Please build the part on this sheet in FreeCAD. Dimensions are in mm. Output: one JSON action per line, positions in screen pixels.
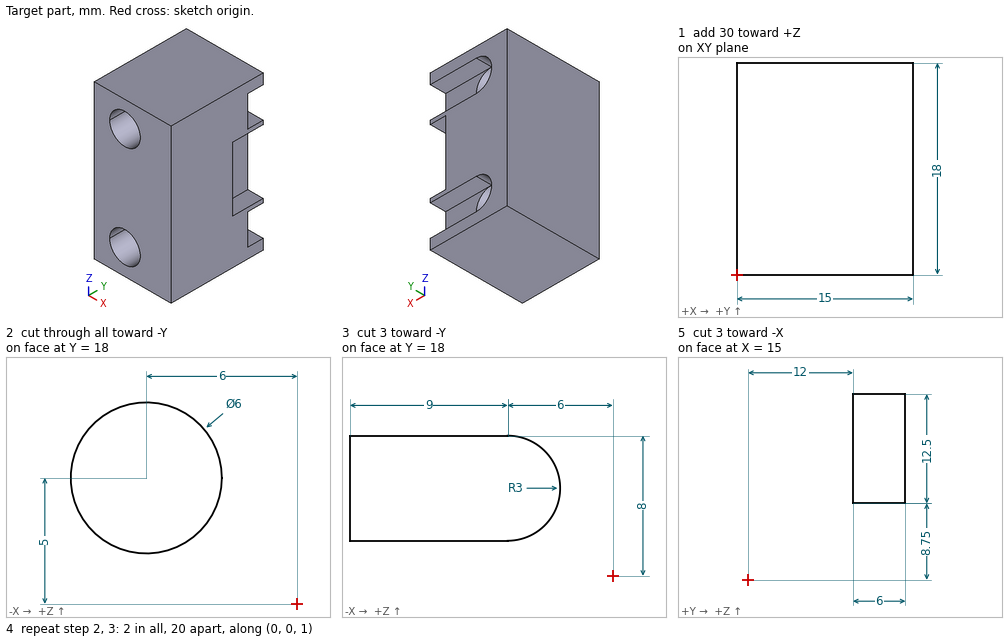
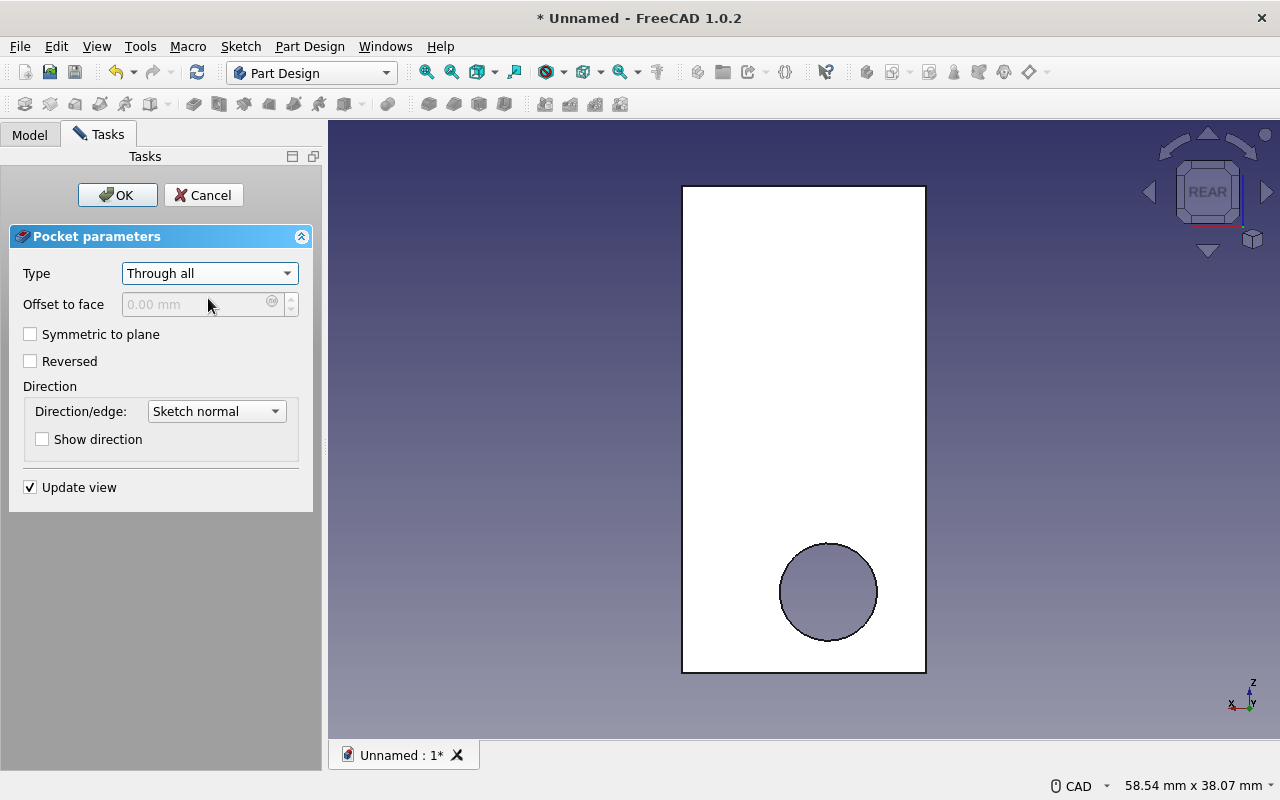
{"action": "left_click", "coordinate": [118, 195]}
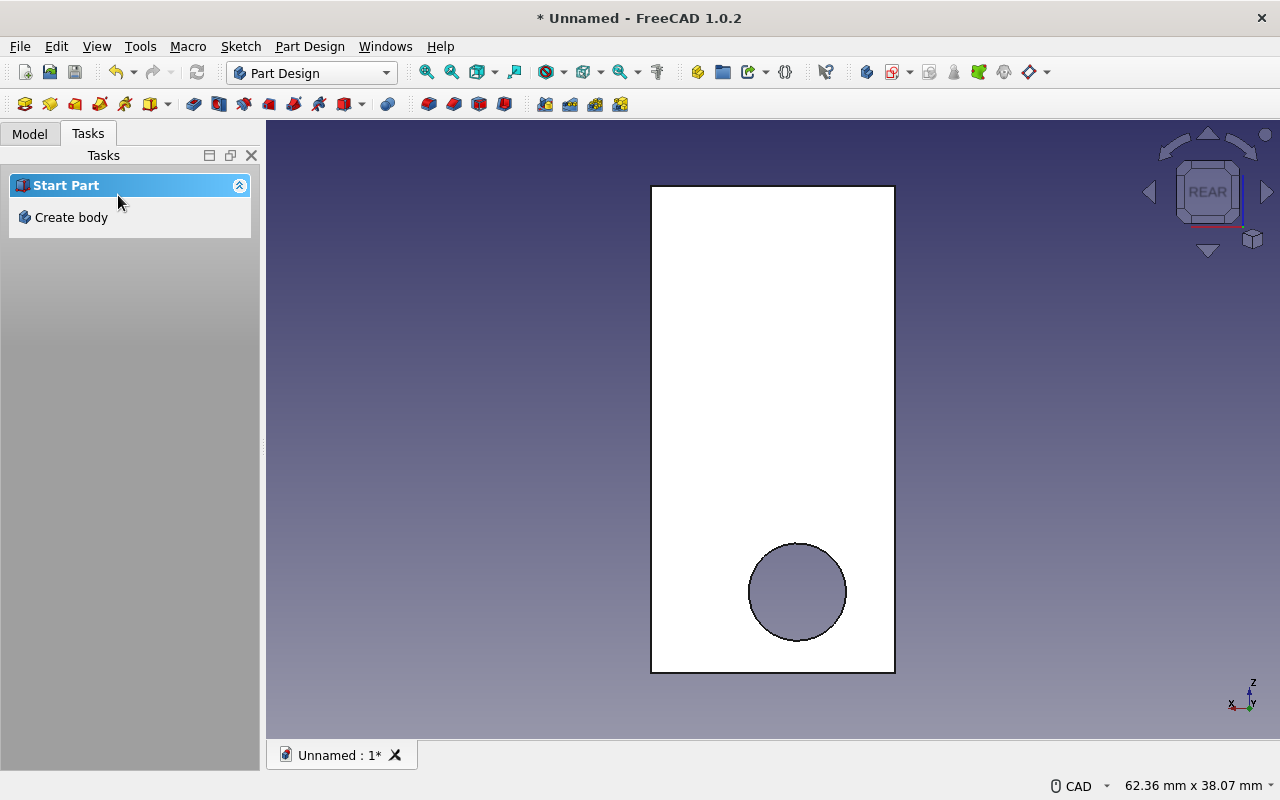
{"action": "left_click", "coordinate": [773, 359]}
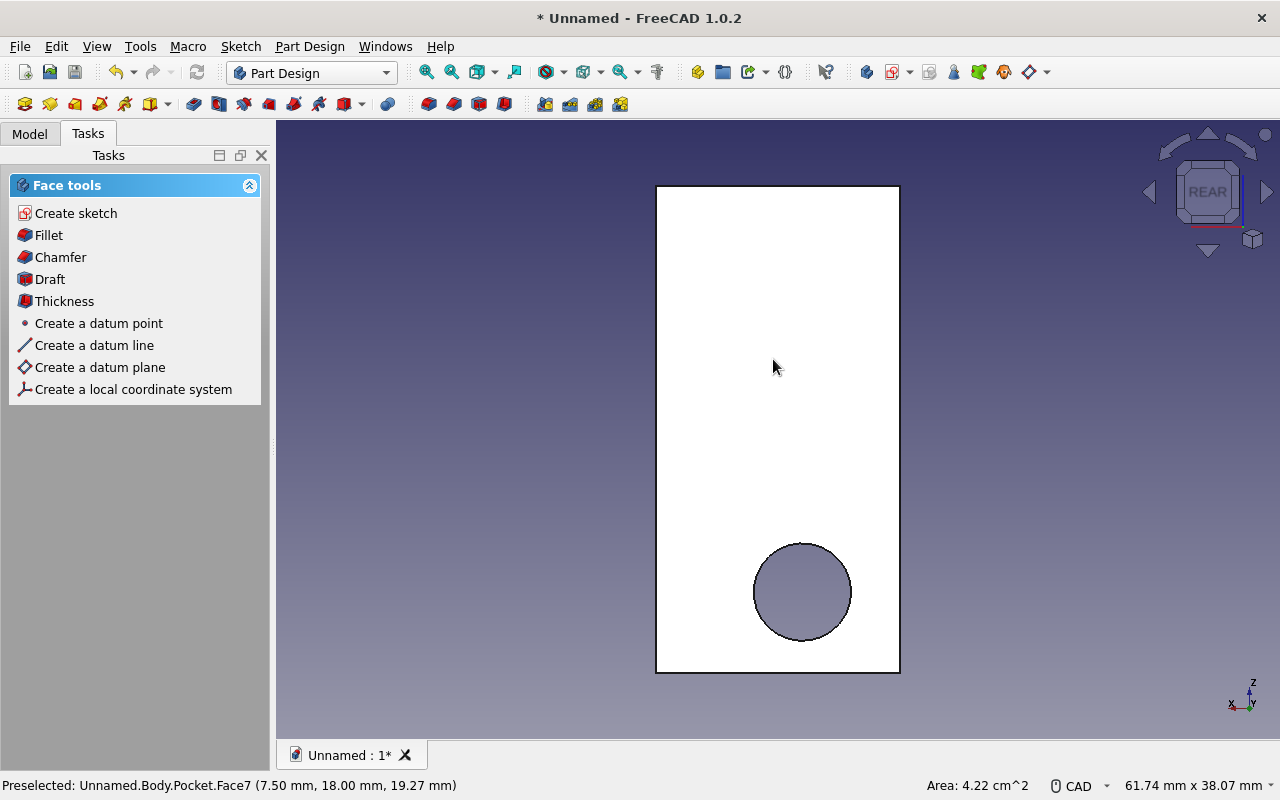
{"action": "left_click", "coordinate": [892, 72]}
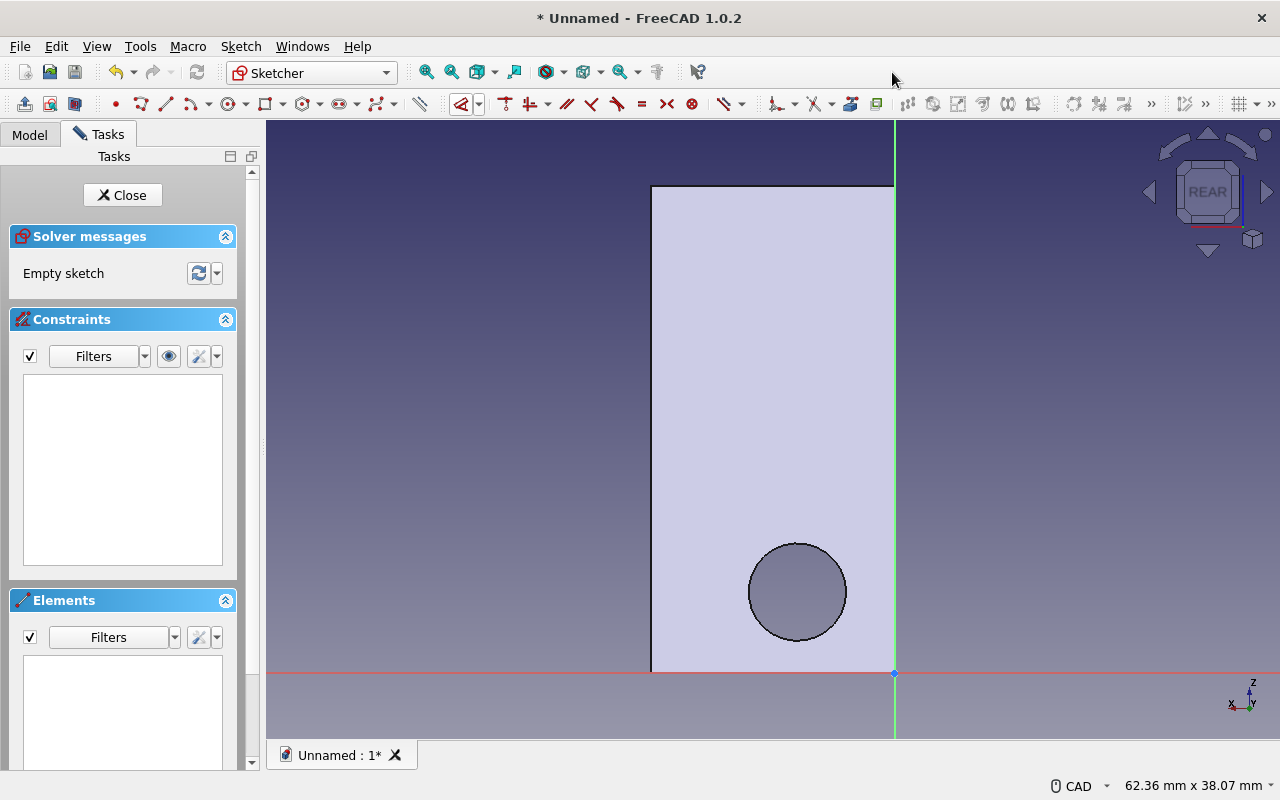
{"action": "scroll", "coordinate": [829, 711], "scroll_direction": "up", "scroll_amount": 4}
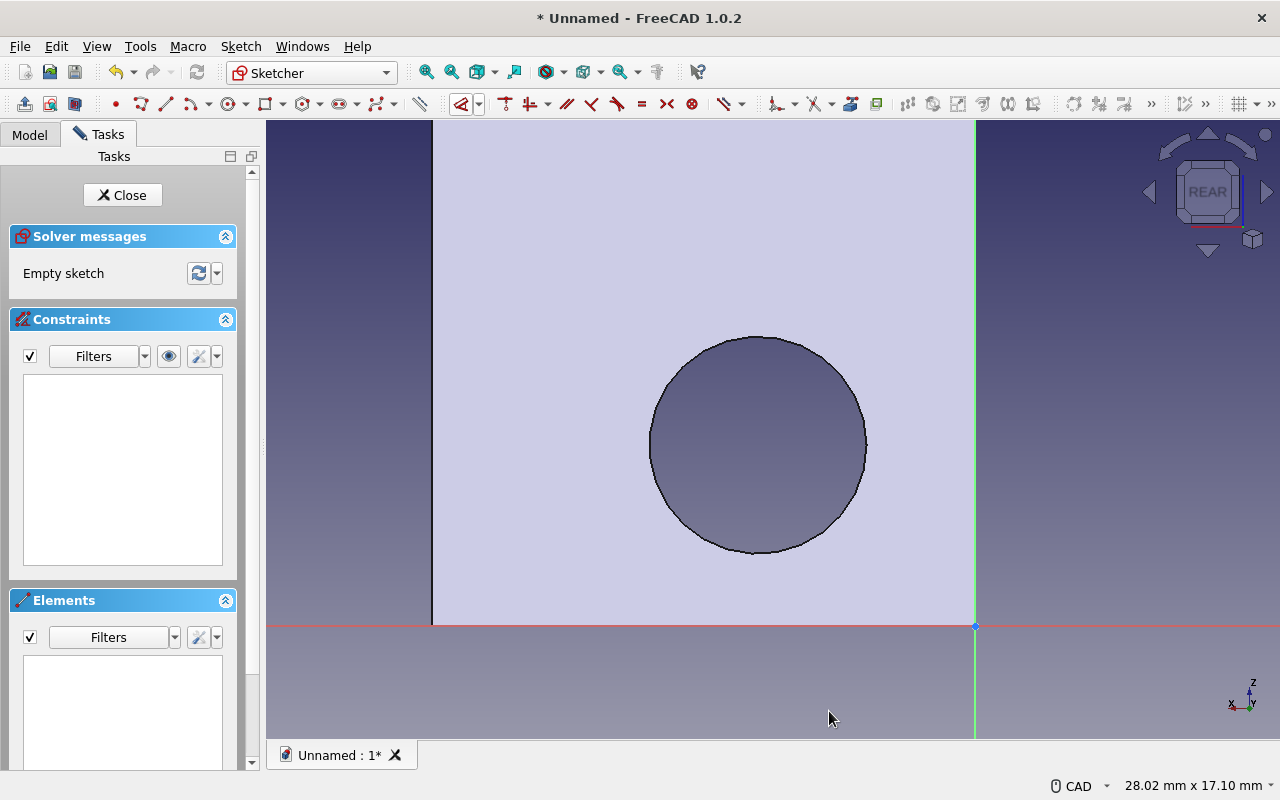
{"action": "left_click", "coordinate": [141, 104]}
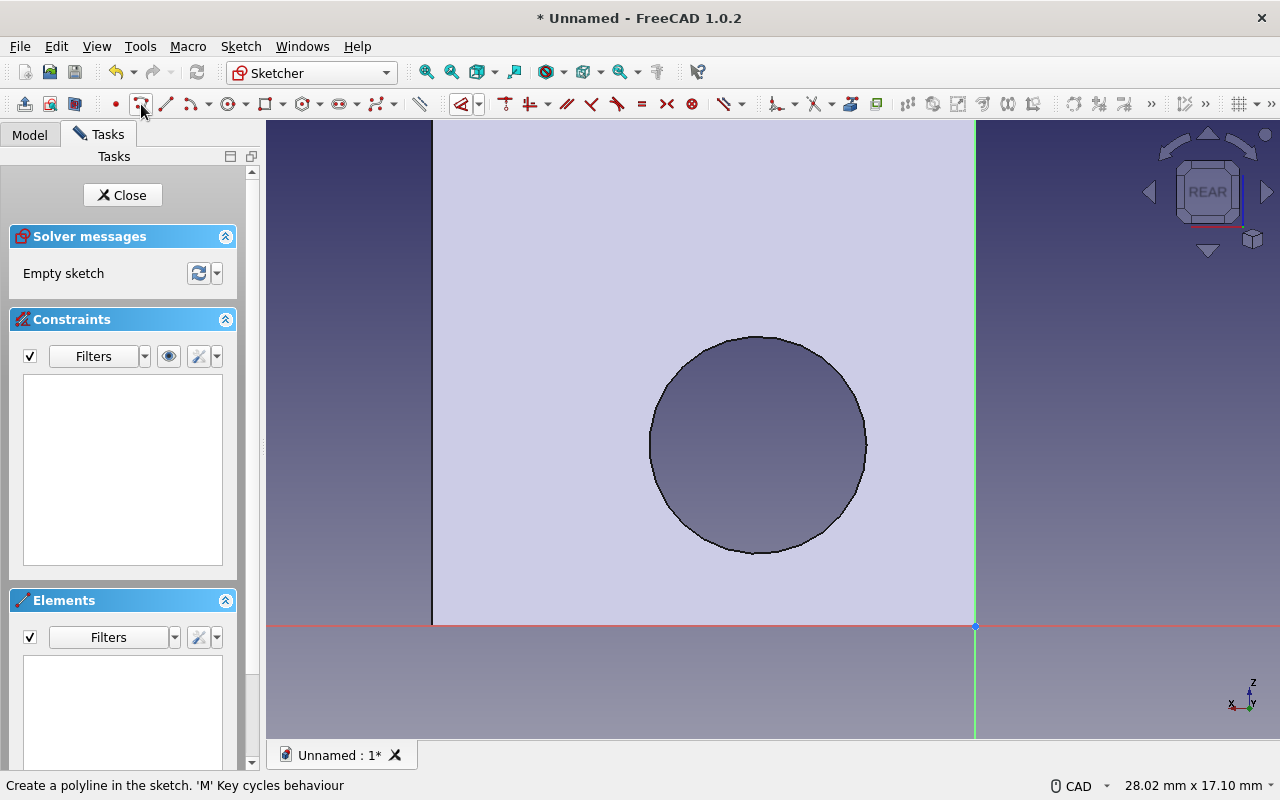
{"action": "left_click", "coordinate": [758, 337]}
{"action": "left_click", "coordinate": [432, 337]}
{"action": "left_click", "coordinate": [432, 554]}
{"action": "left_click", "coordinate": [758, 554]}
{"action": "right_click", "coordinate": [758, 554]}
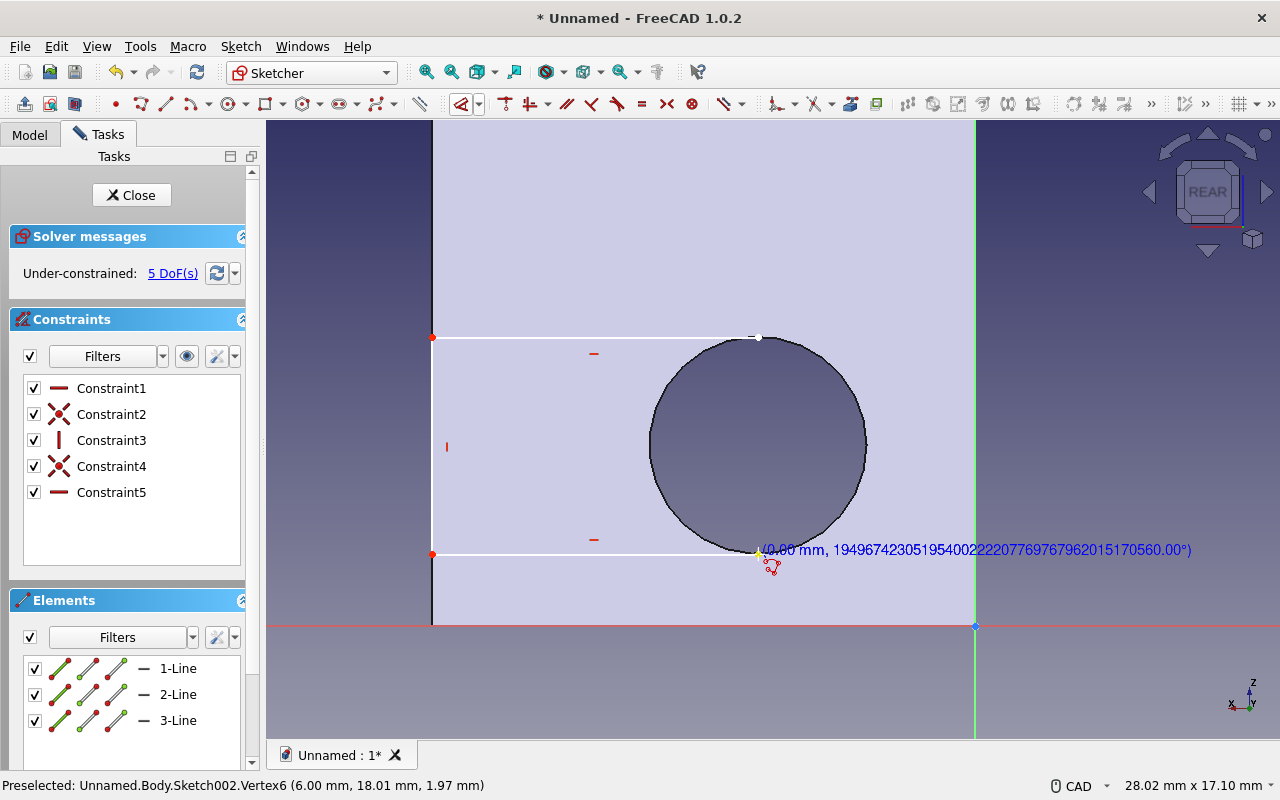
{"action": "key", "text": "g 3 a"}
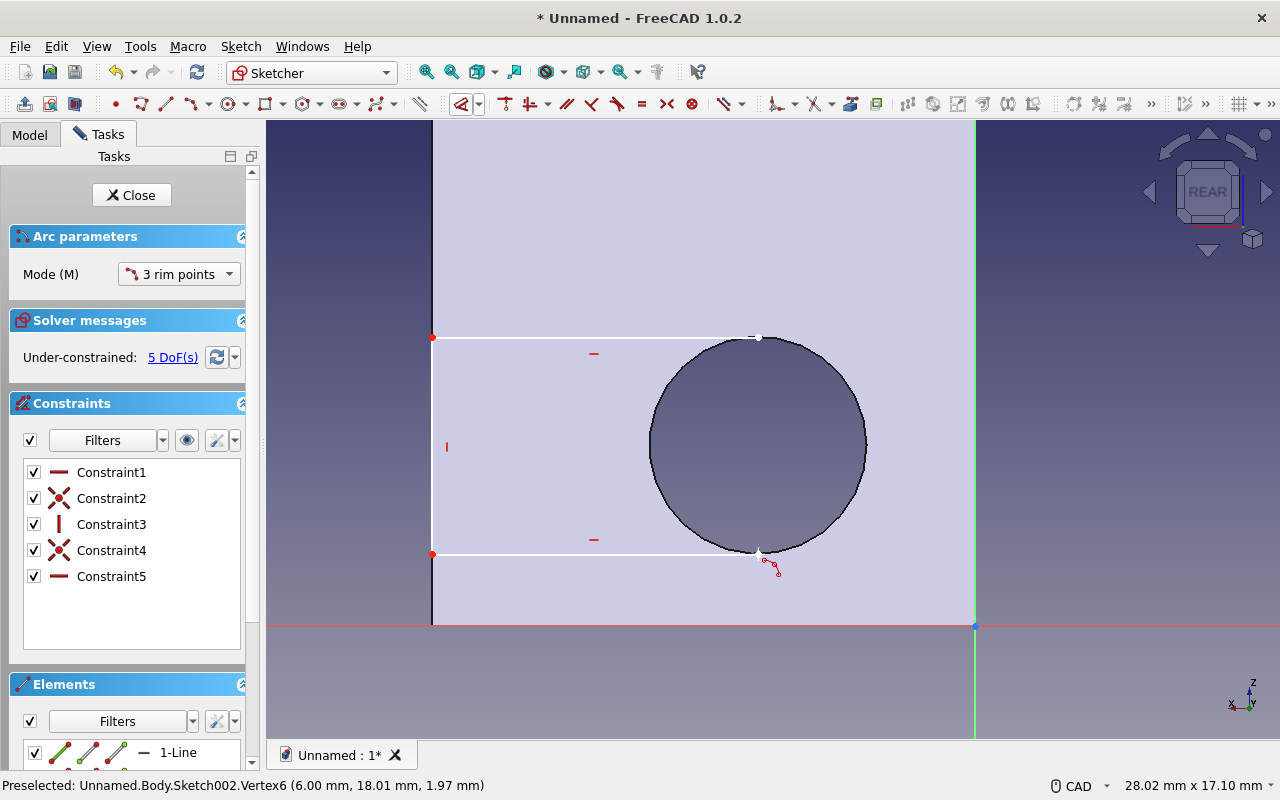
{"action": "left_click", "coordinate": [758, 555]}
{"action": "left_click", "coordinate": [758, 338]}
{"action": "left_click", "coordinate": [867, 445]}
{"action": "key", "text": "Escape"}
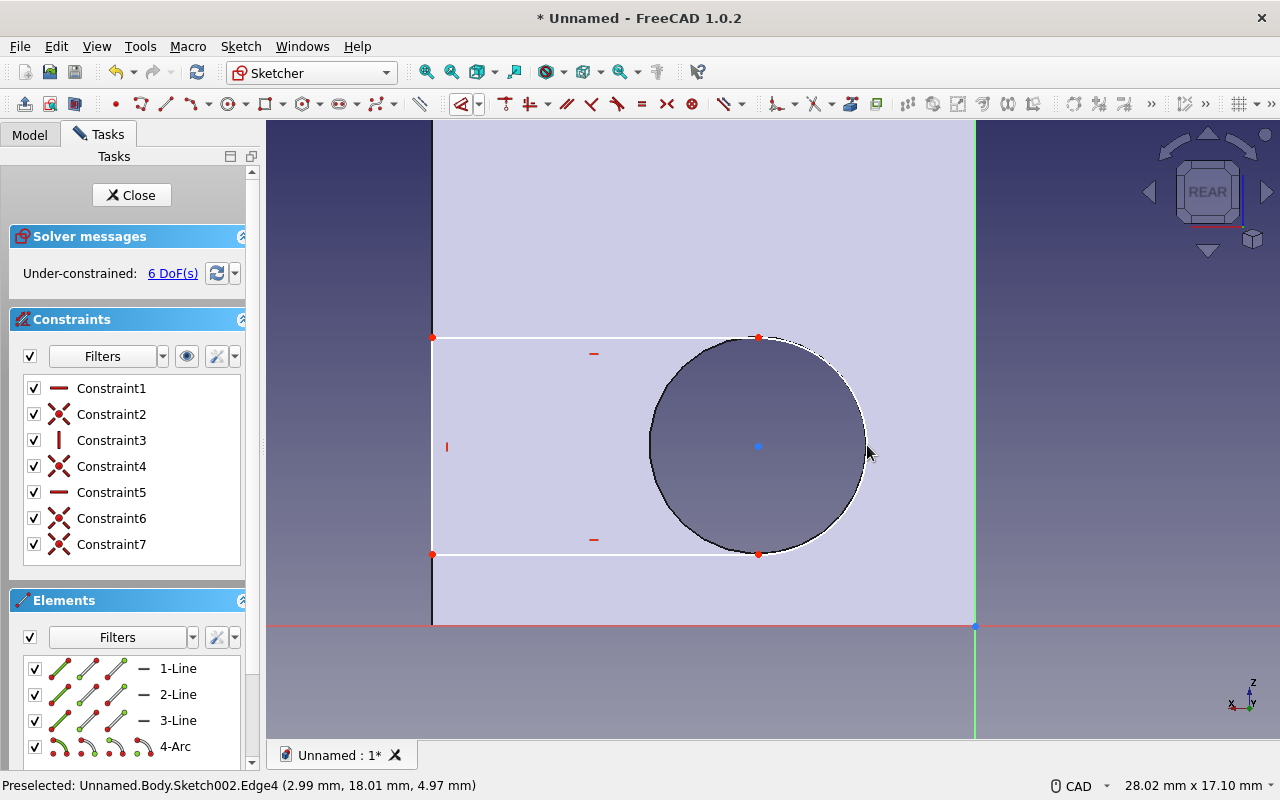
{"action": "left_click", "coordinate": [660, 338]}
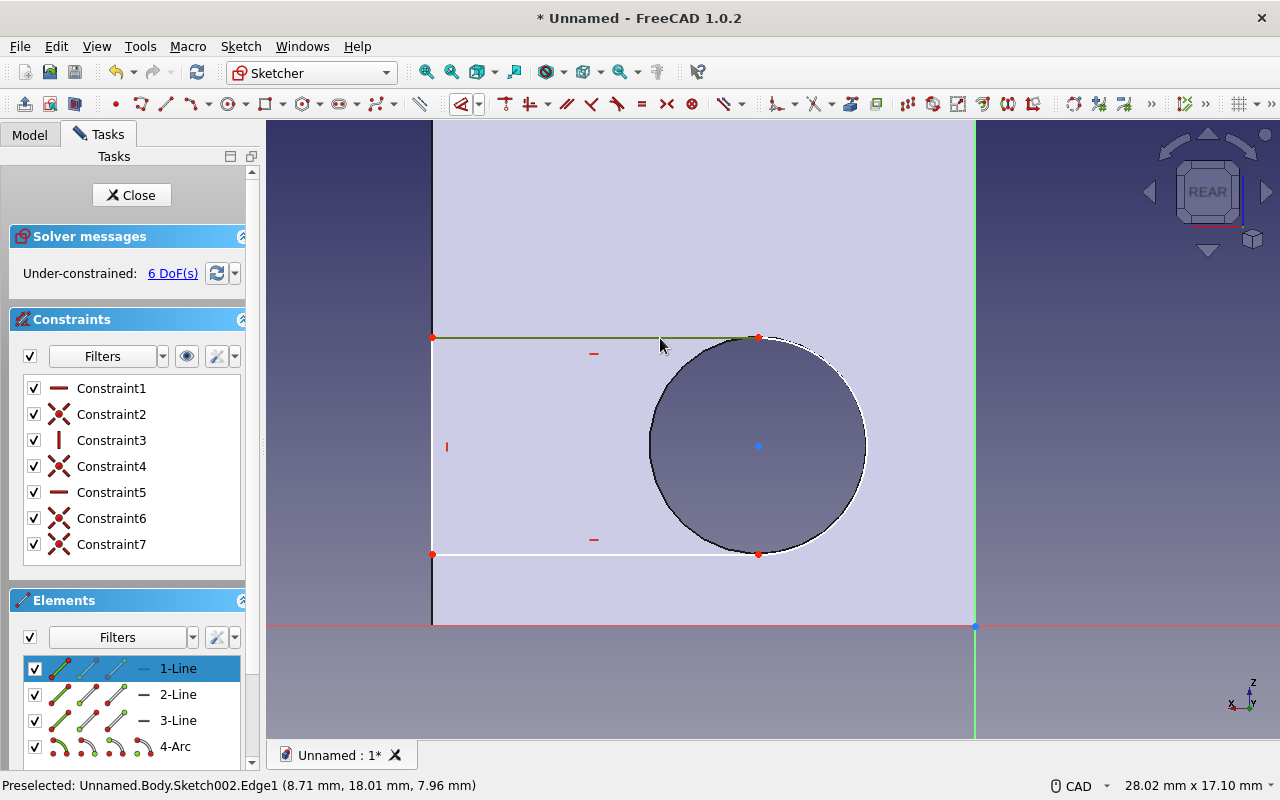
{"action": "left_click", "coordinate": [846, 510]}